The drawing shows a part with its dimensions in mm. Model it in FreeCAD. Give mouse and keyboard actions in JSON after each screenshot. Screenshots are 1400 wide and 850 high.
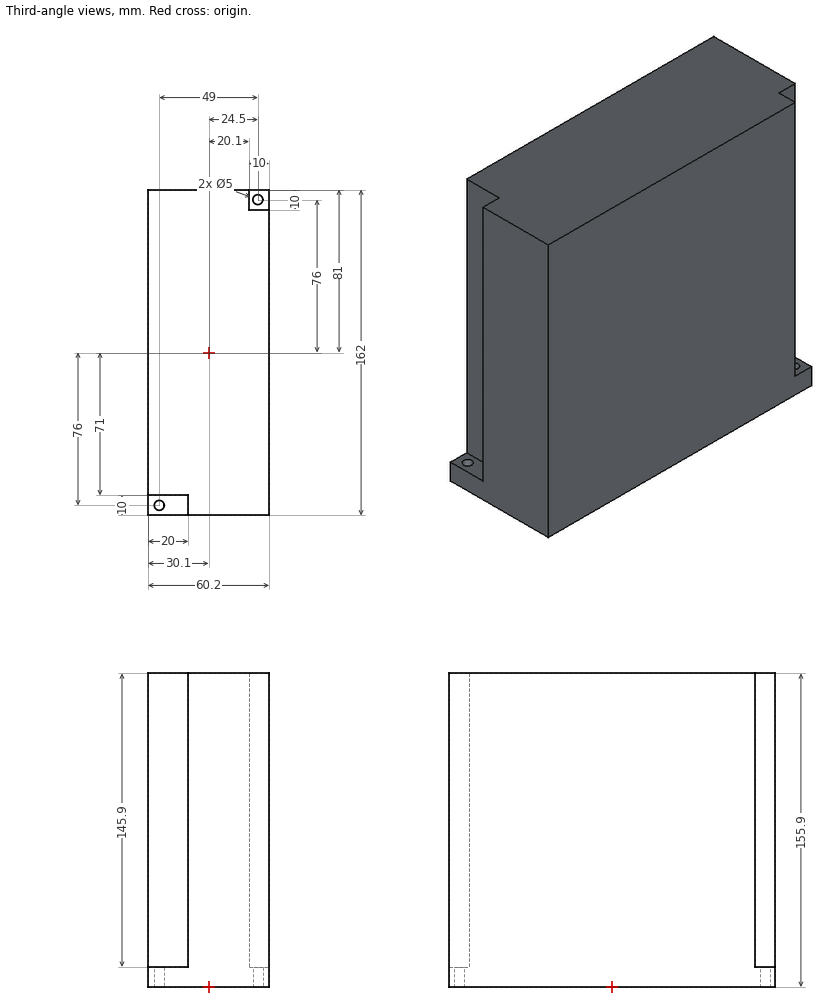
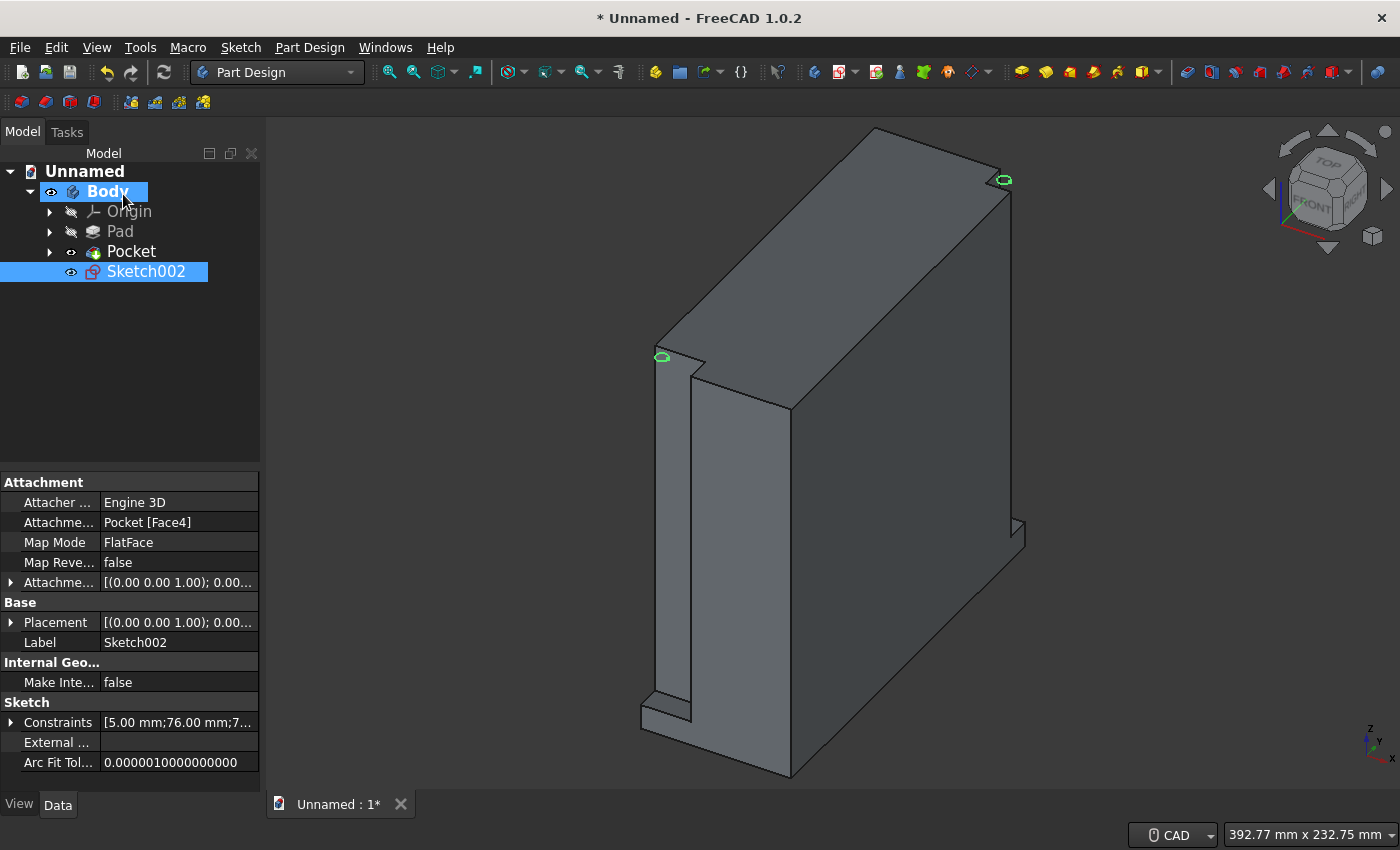
{"action": "left_click", "coordinate": [1188, 72]}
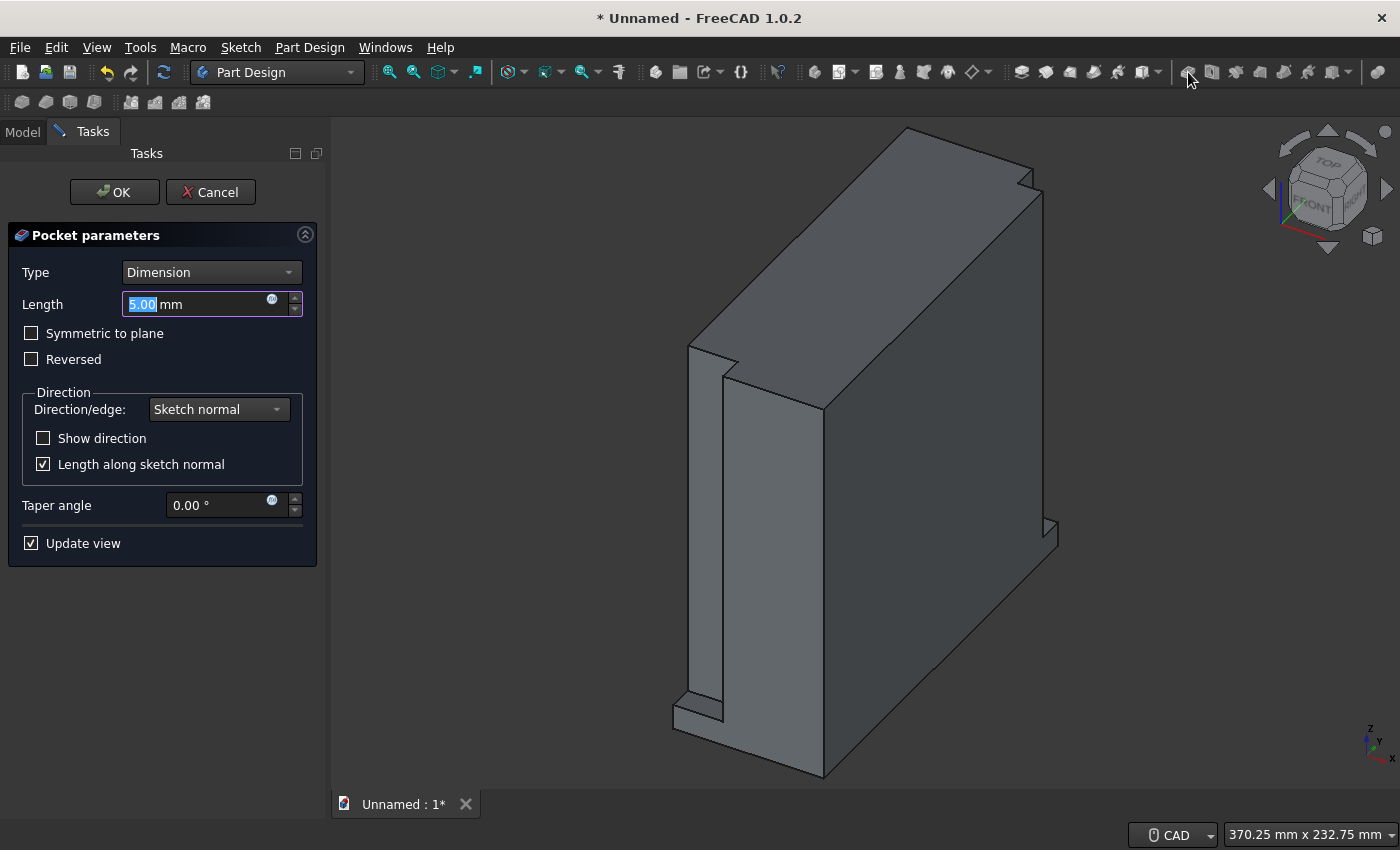
{"action": "left_click", "coordinate": [212, 272]}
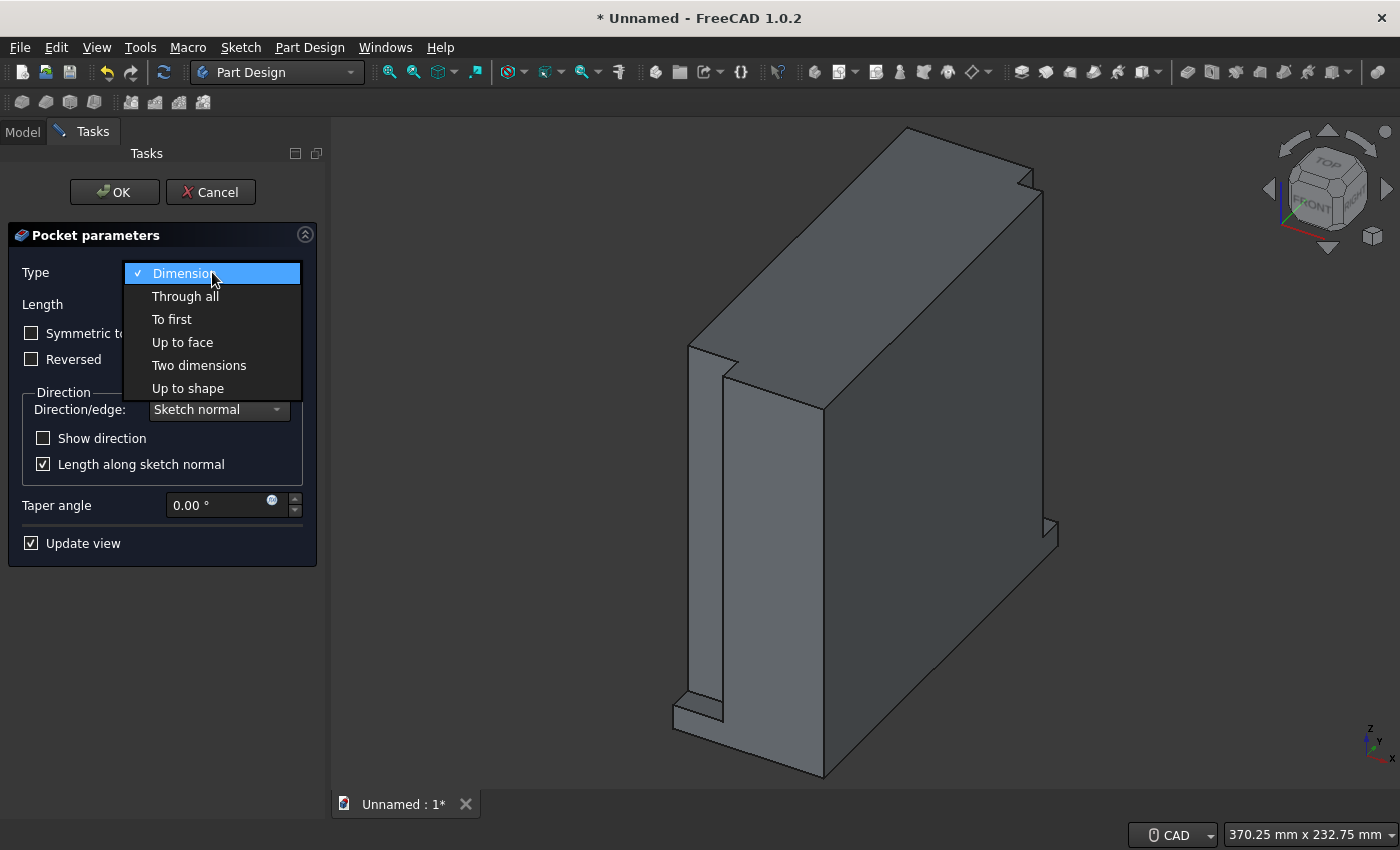
{"action": "left_click", "coordinate": [212, 296]}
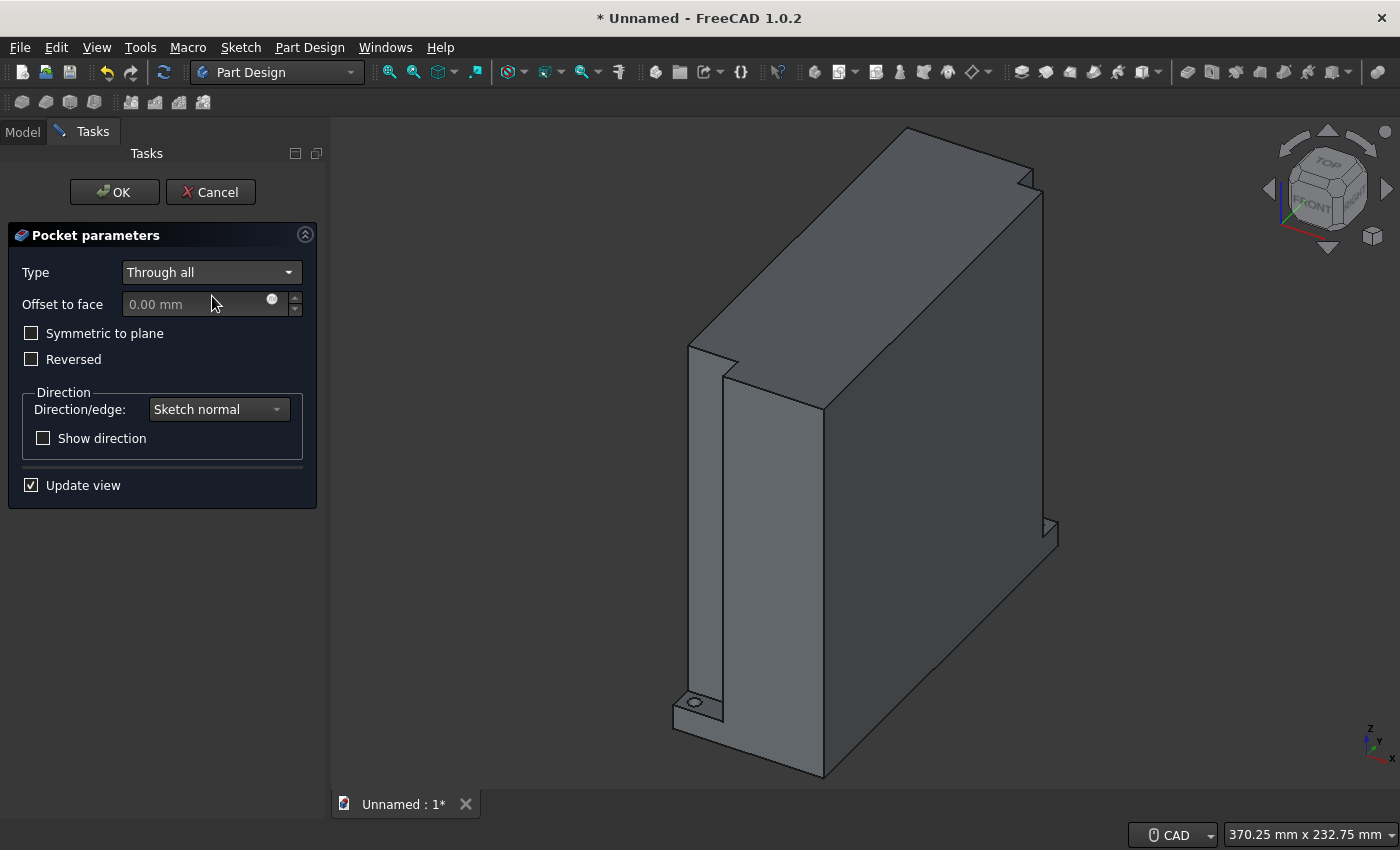
{"action": "left_click", "coordinate": [115, 192]}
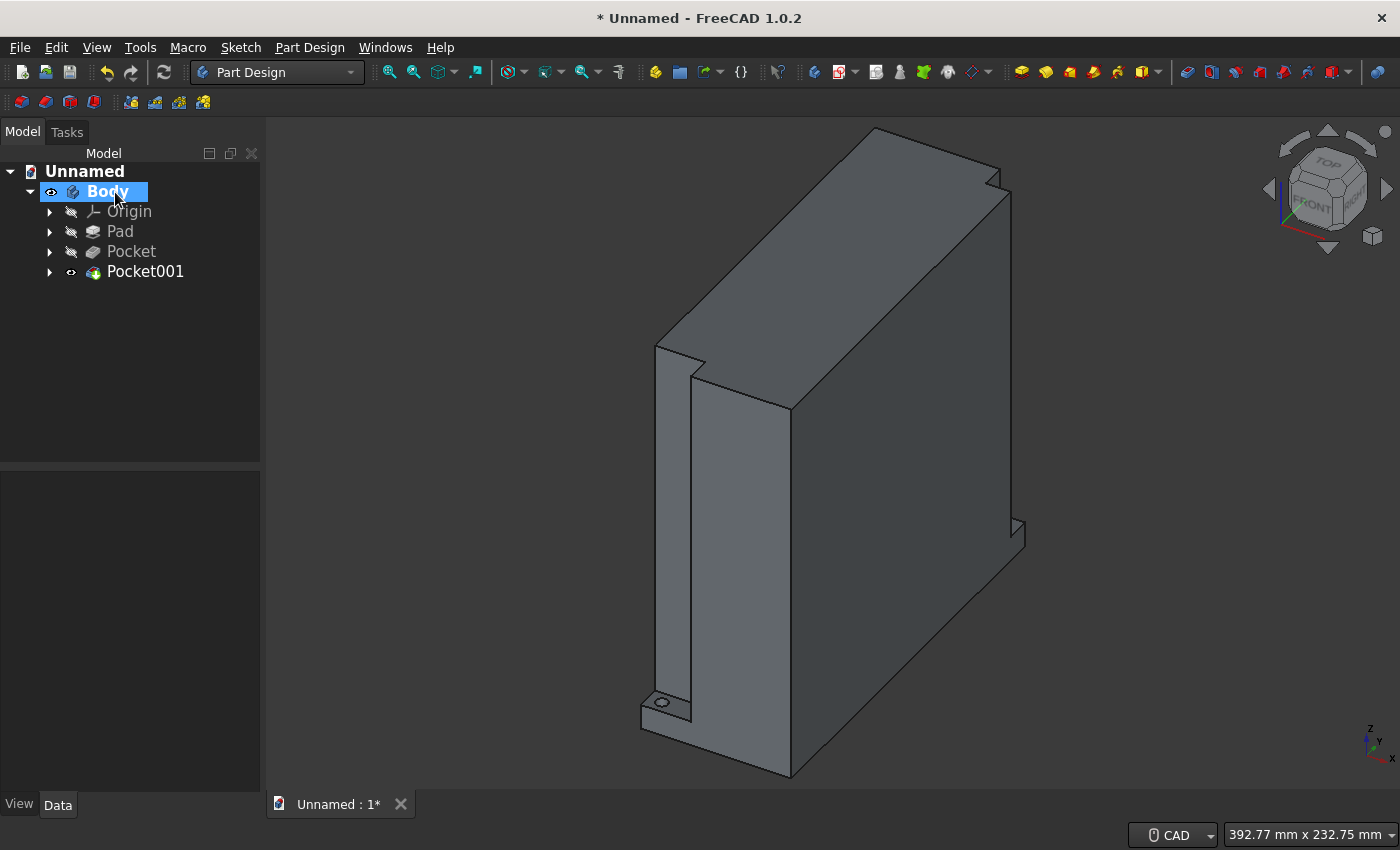
{"action": "key", "text": "0"}